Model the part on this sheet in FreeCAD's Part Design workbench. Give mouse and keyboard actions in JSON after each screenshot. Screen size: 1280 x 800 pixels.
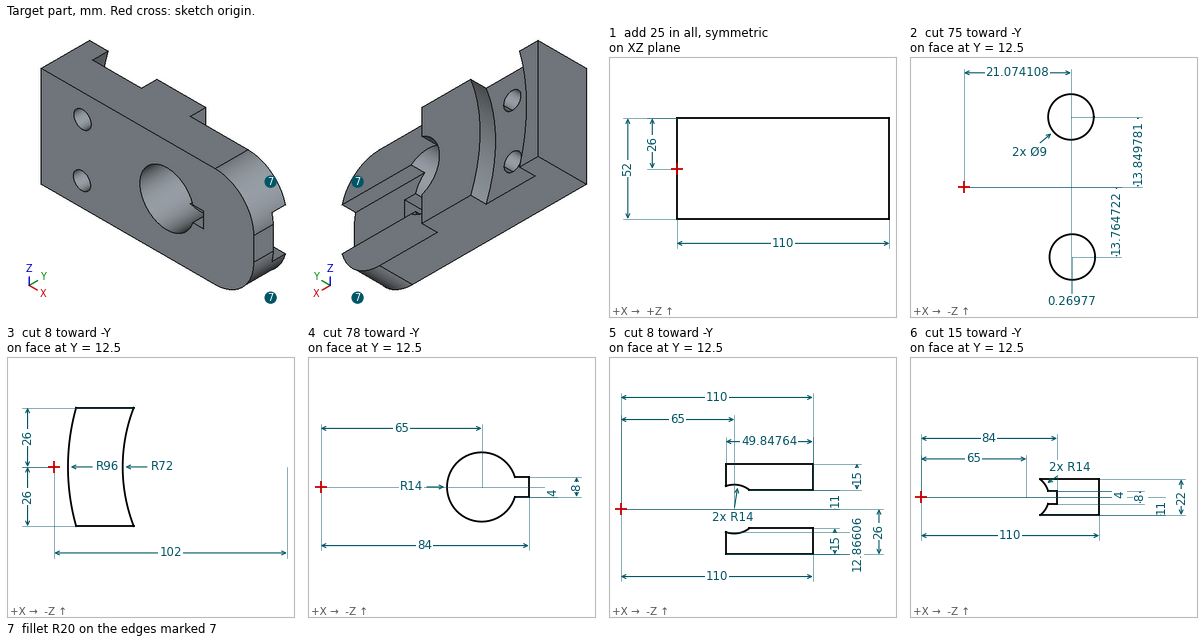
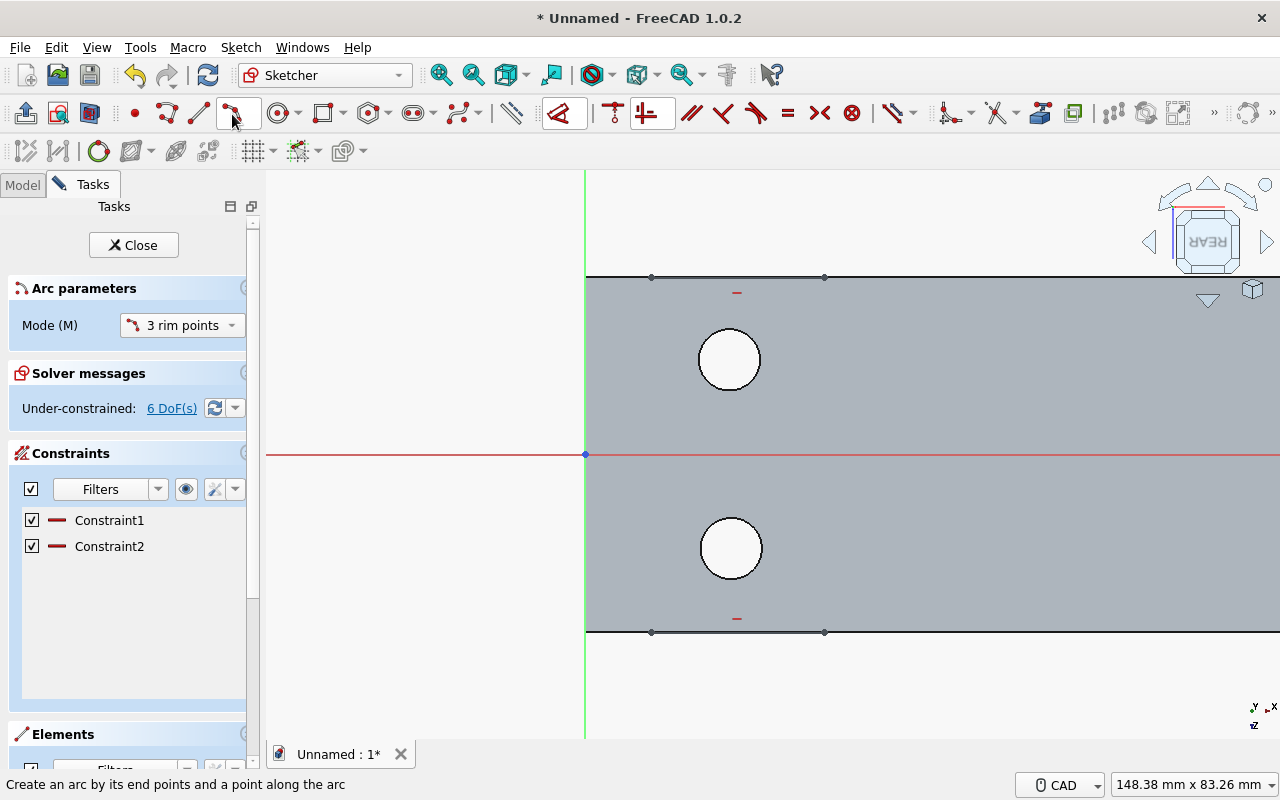
{"action": "left_click", "coordinate": [651, 278]}
{"action": "left_click", "coordinate": [651, 633]}
{"action": "left_click", "coordinate": [627, 419]}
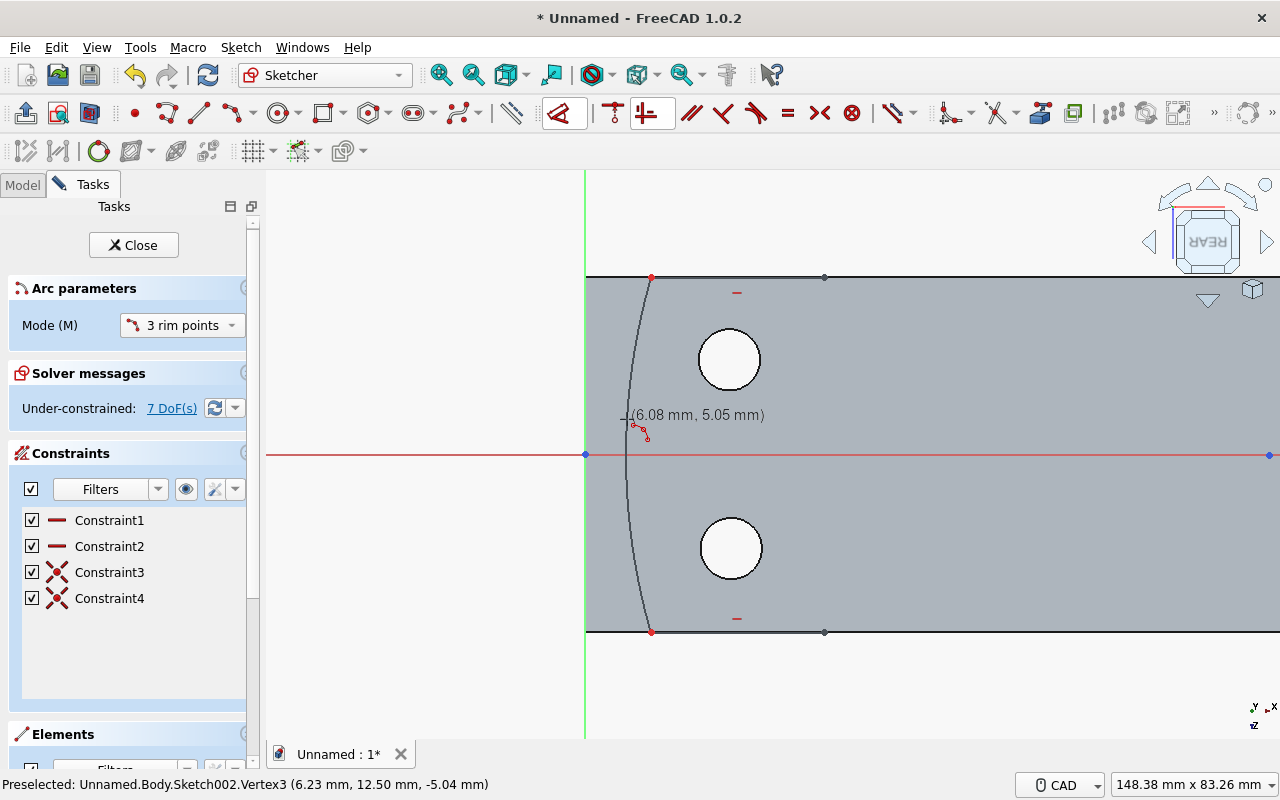
{"action": "left_click", "coordinate": [824, 633]}
{"action": "left_click", "coordinate": [824, 278]}
{"action": "left_click", "coordinate": [792, 418]}
{"action": "key", "text": "Escape"}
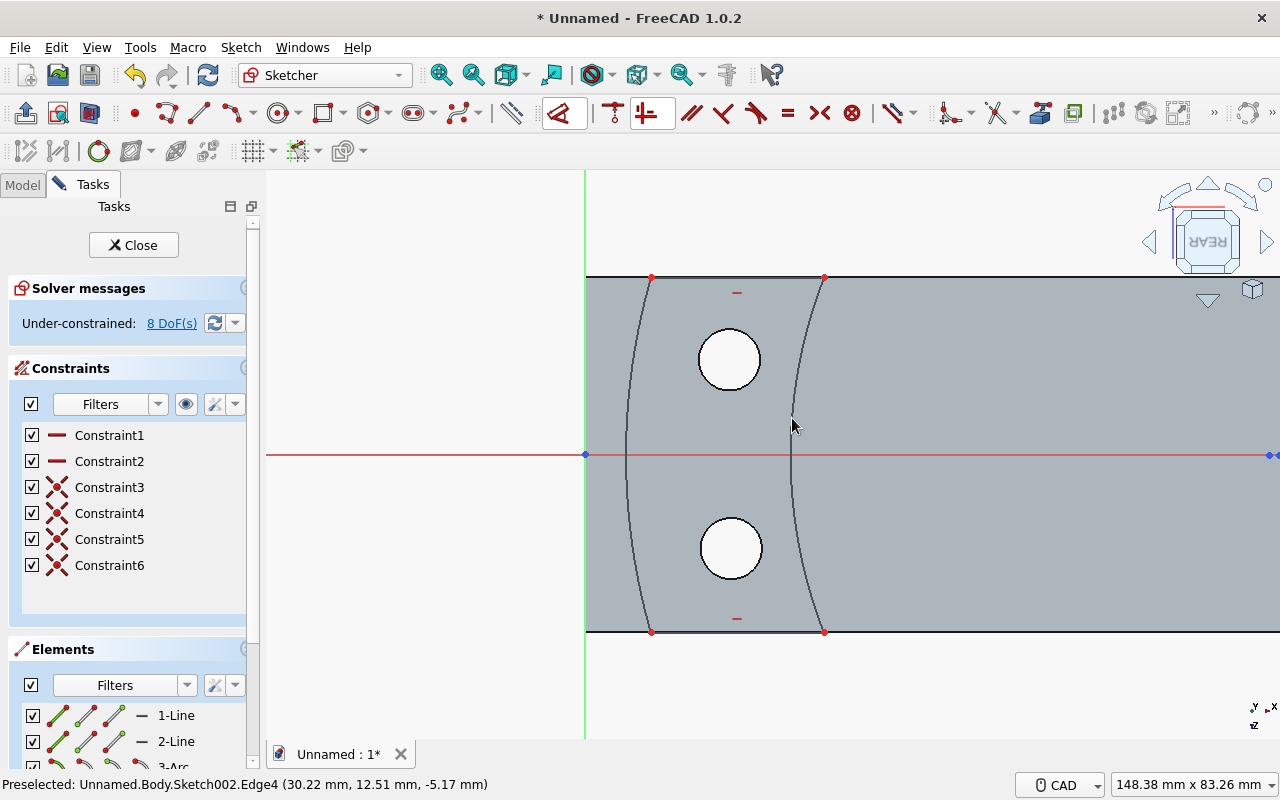
{"action": "left_click", "coordinate": [630, 384]}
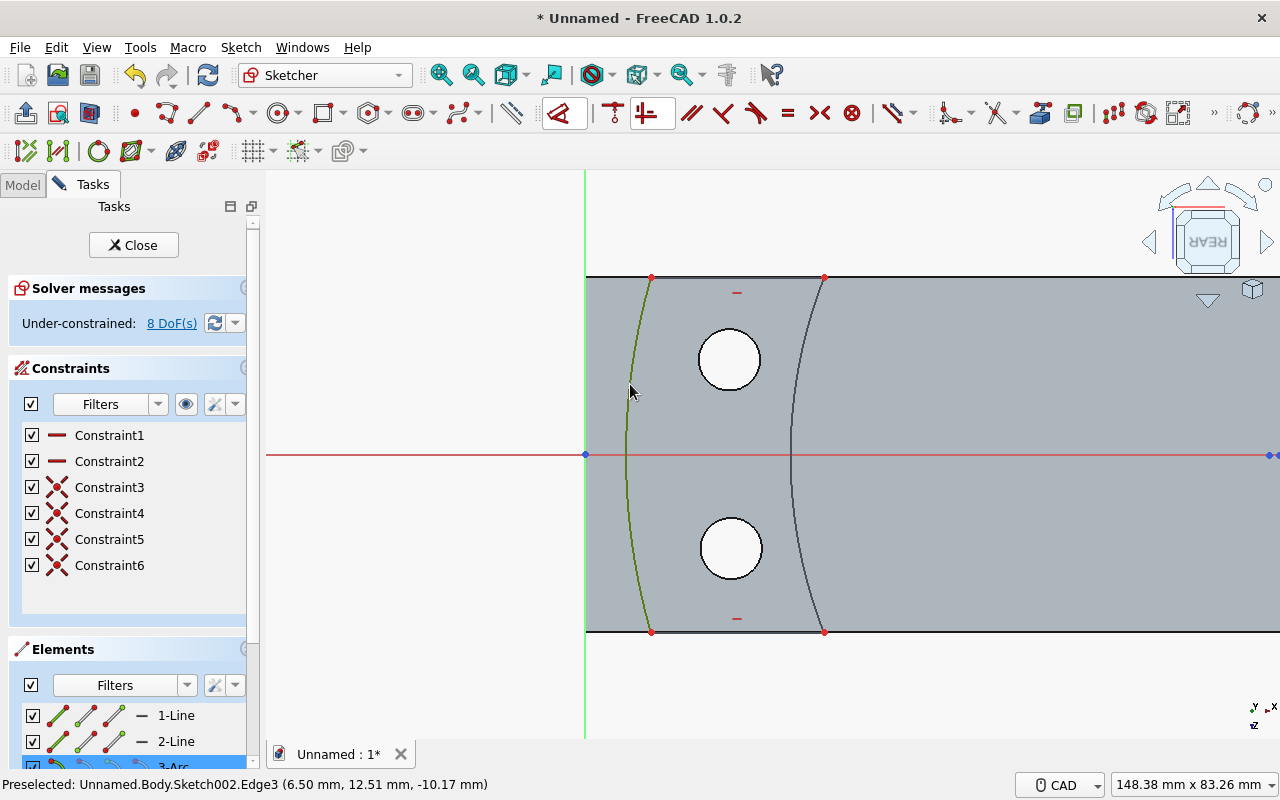
{"action": "left_click", "coordinate": [796, 383]}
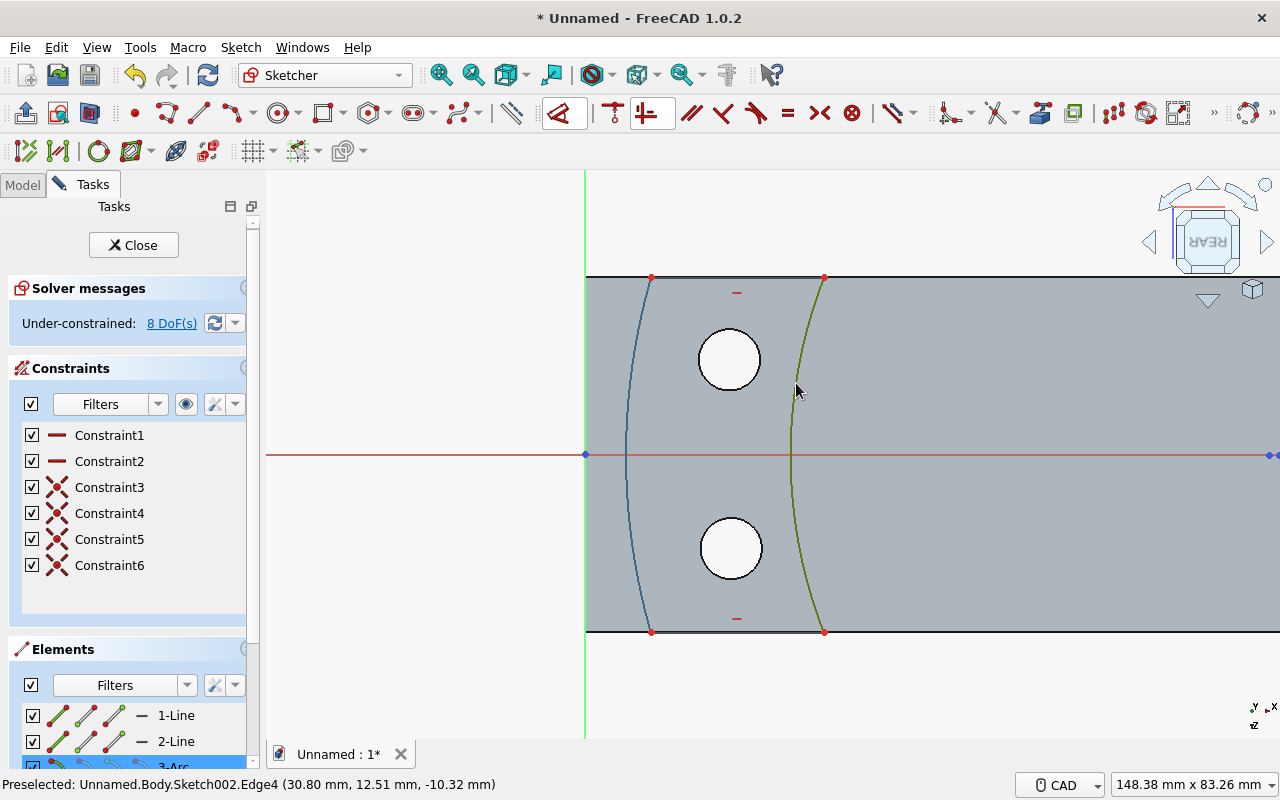
{"action": "left_click", "coordinate": [614, 114]}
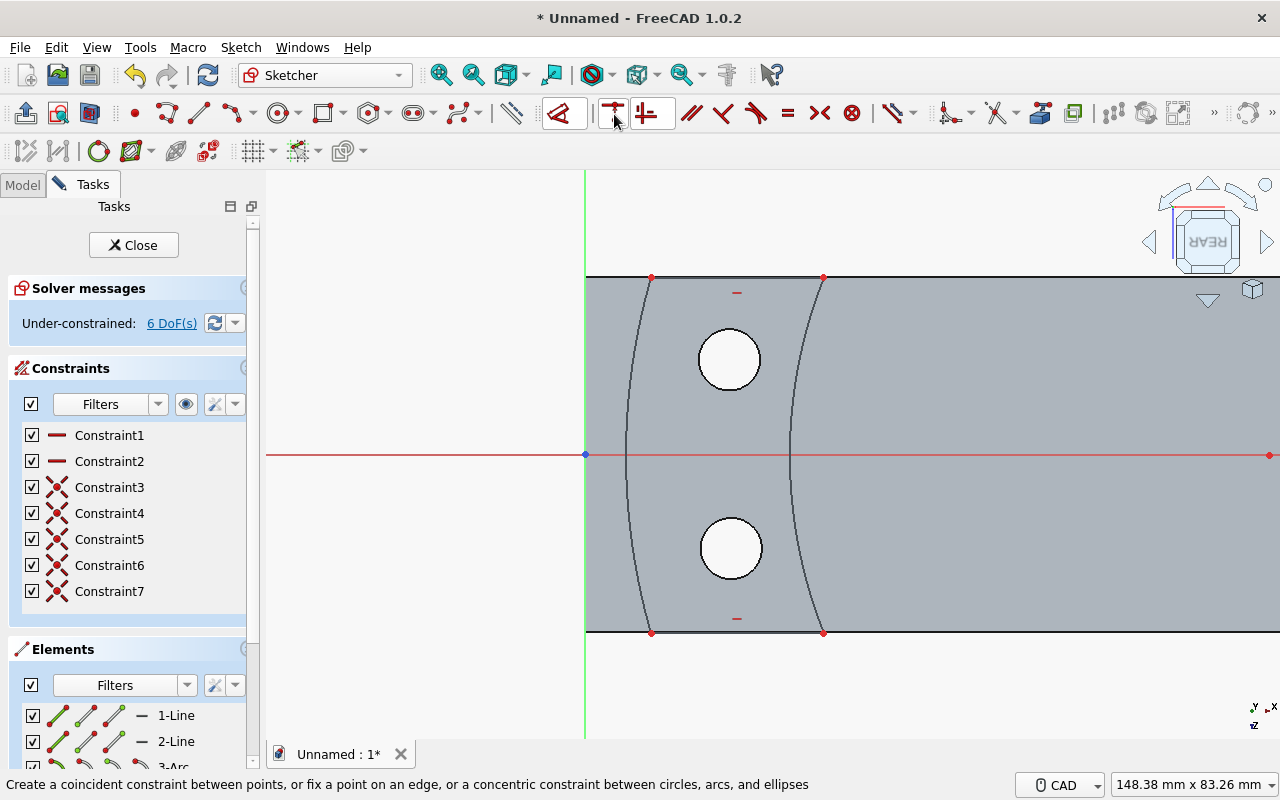
{"action": "scroll", "coordinate": [294, 455], "scroll_direction": "down", "scroll_amount": 2}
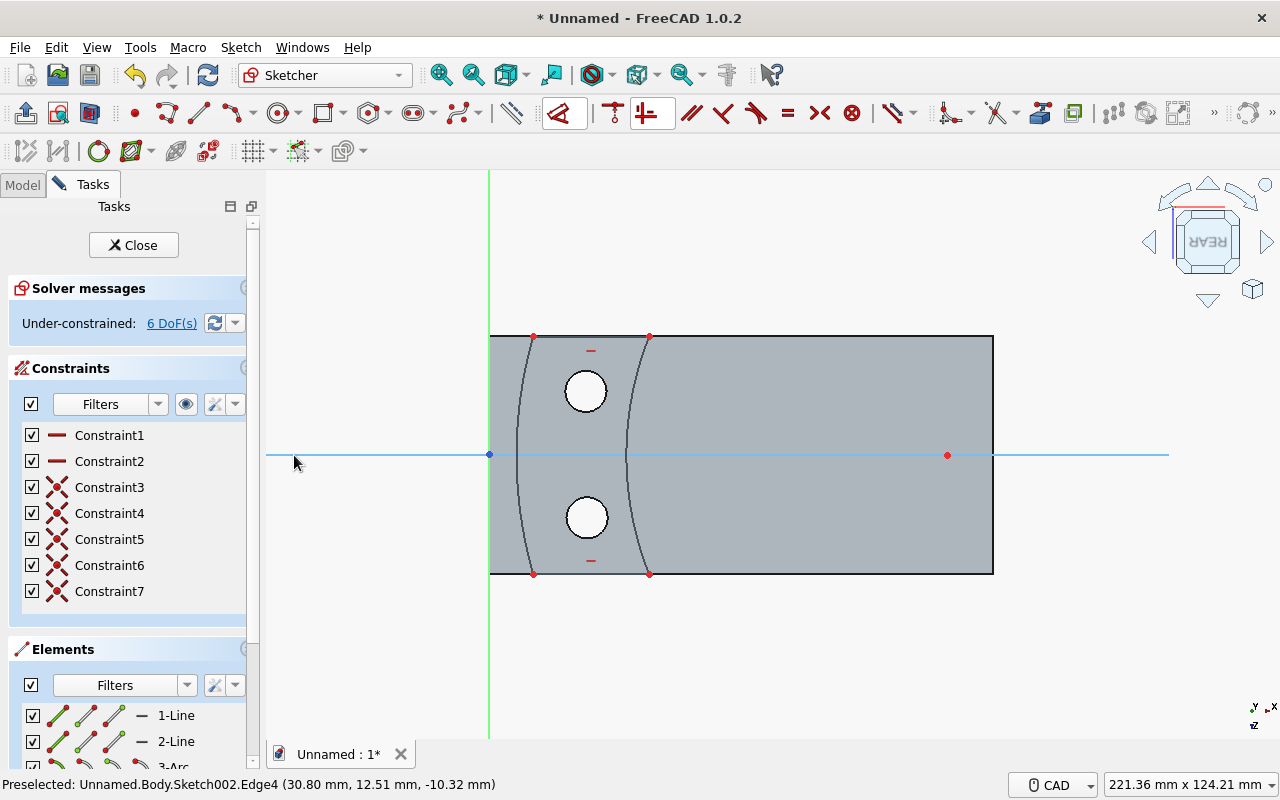
{"action": "left_click", "coordinate": [948, 456]}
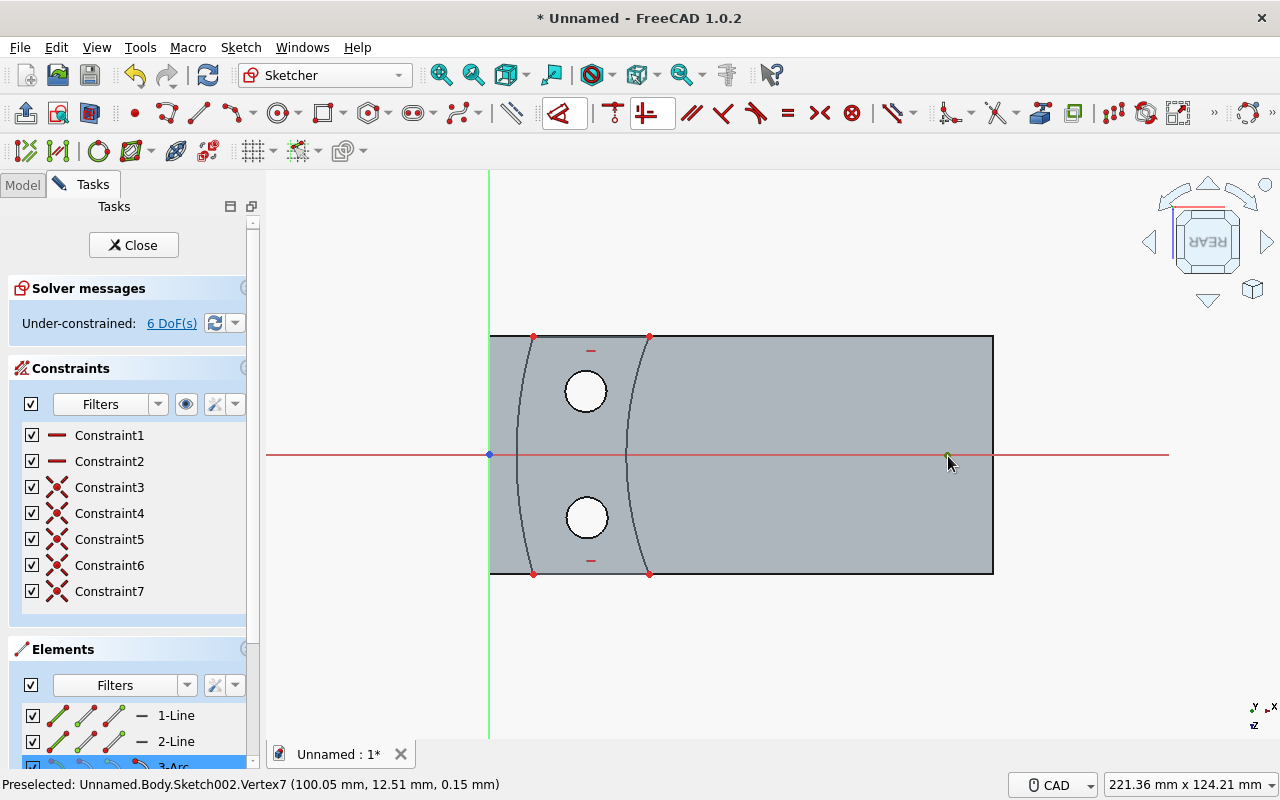
{"action": "left_click", "coordinate": [353, 455]}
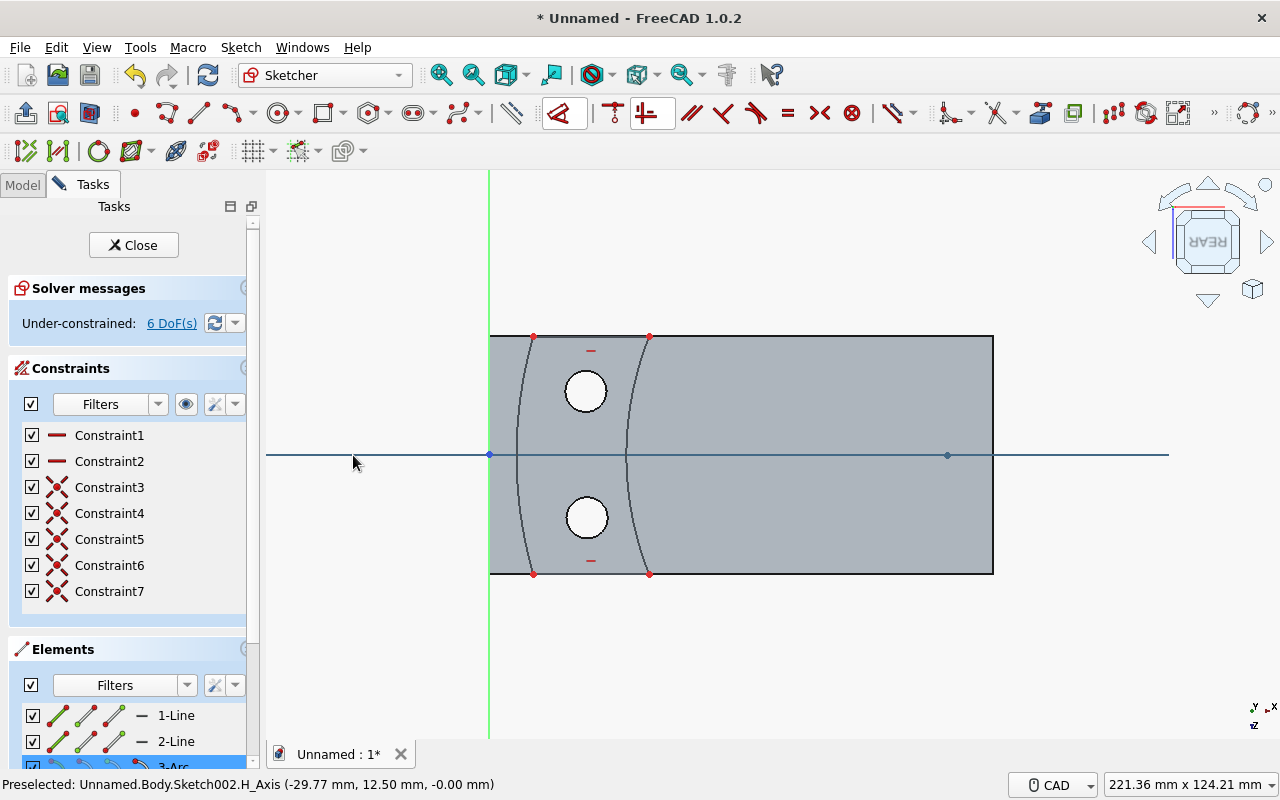
{"action": "left_click", "coordinate": [614, 114]}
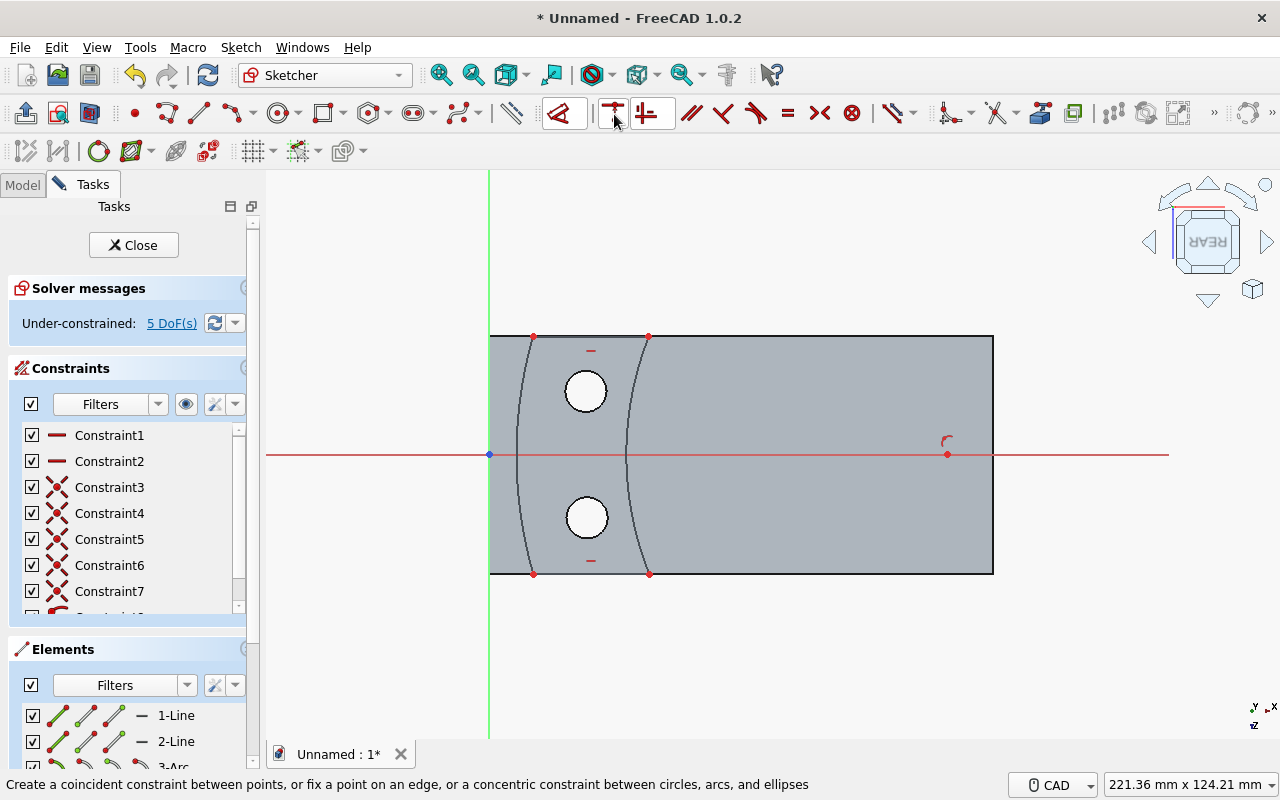
{"action": "left_click", "coordinate": [519, 407]}